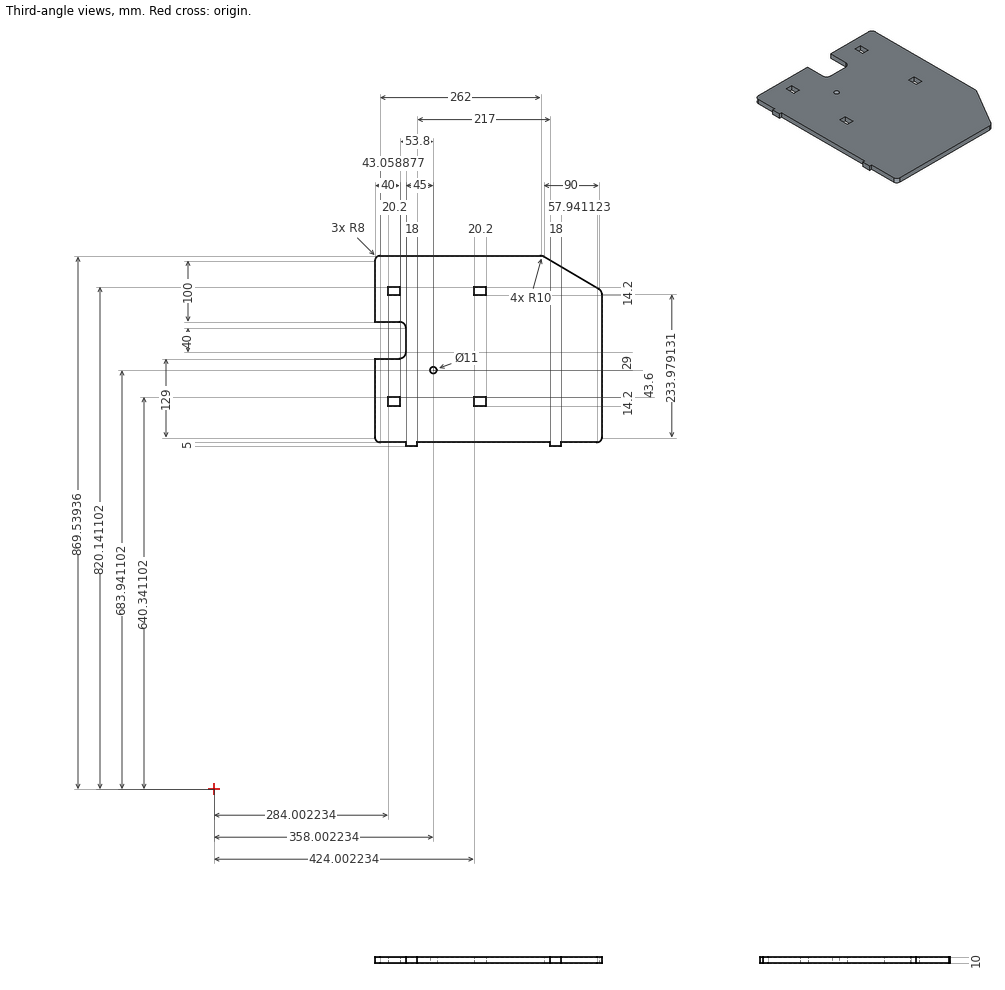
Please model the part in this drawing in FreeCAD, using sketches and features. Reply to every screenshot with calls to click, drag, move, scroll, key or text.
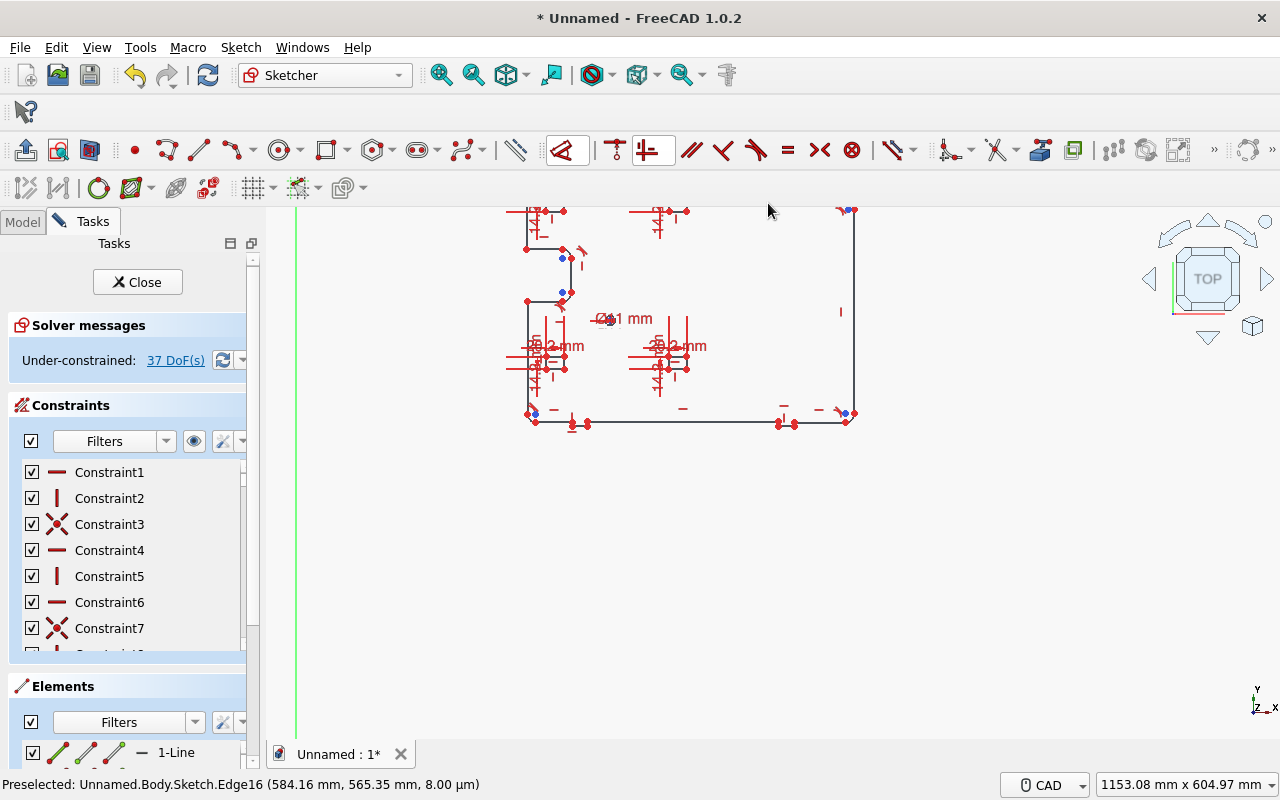
scroll(810, 421, down, 4)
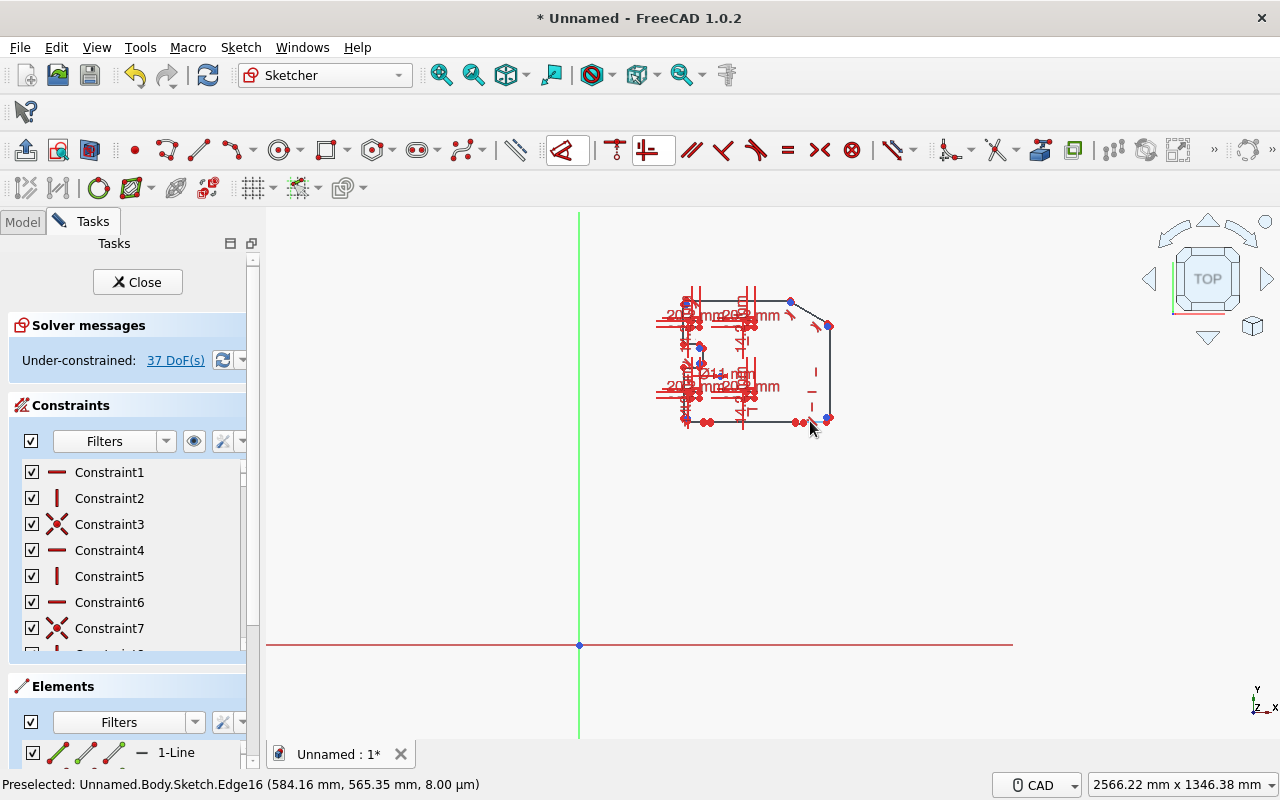
scroll(791, 301, up, 12)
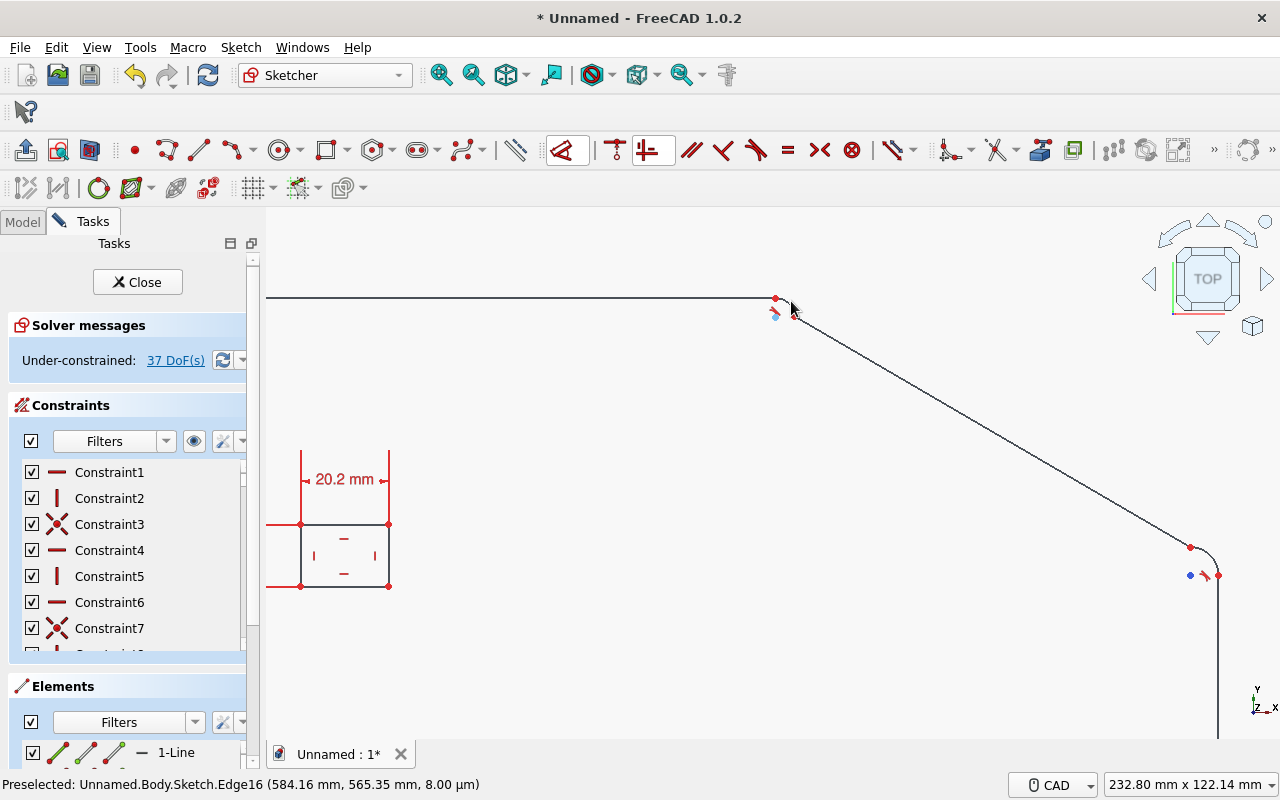
click(789, 303)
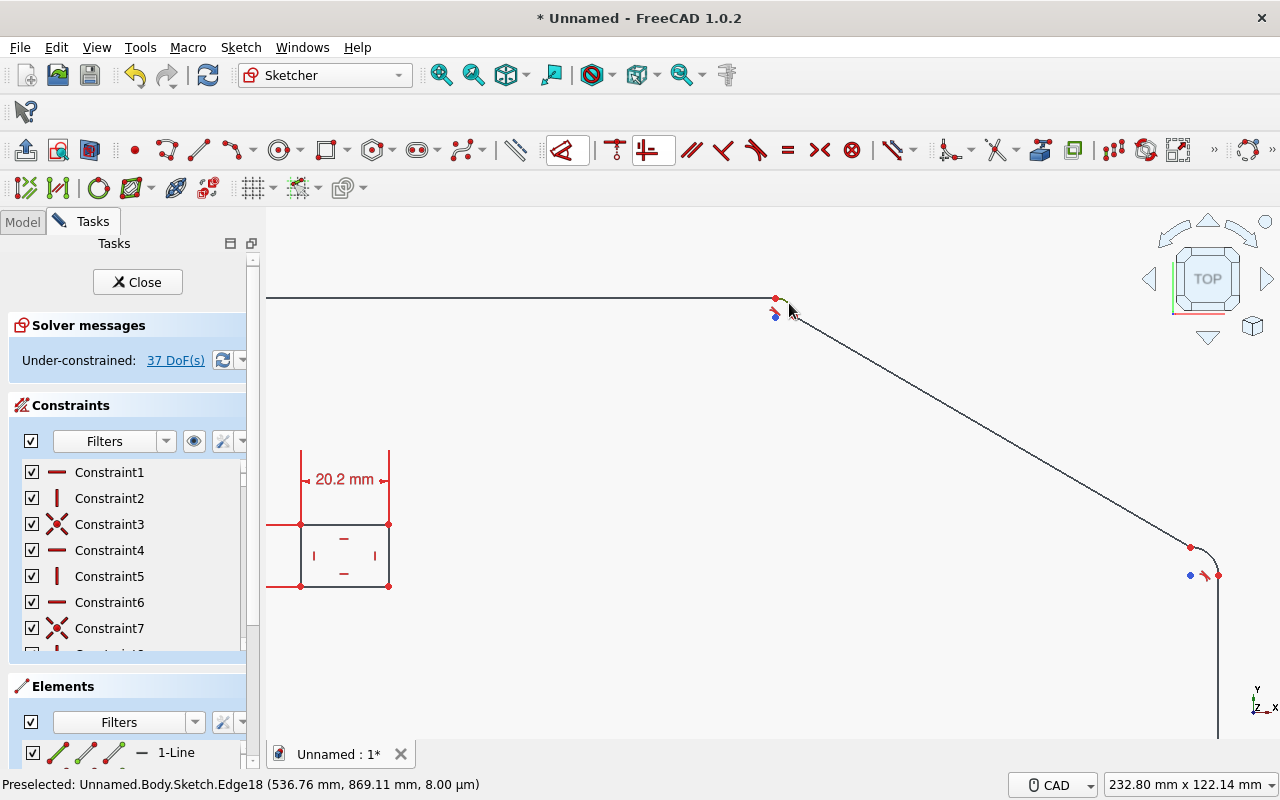
scroll(791, 301, down, 12)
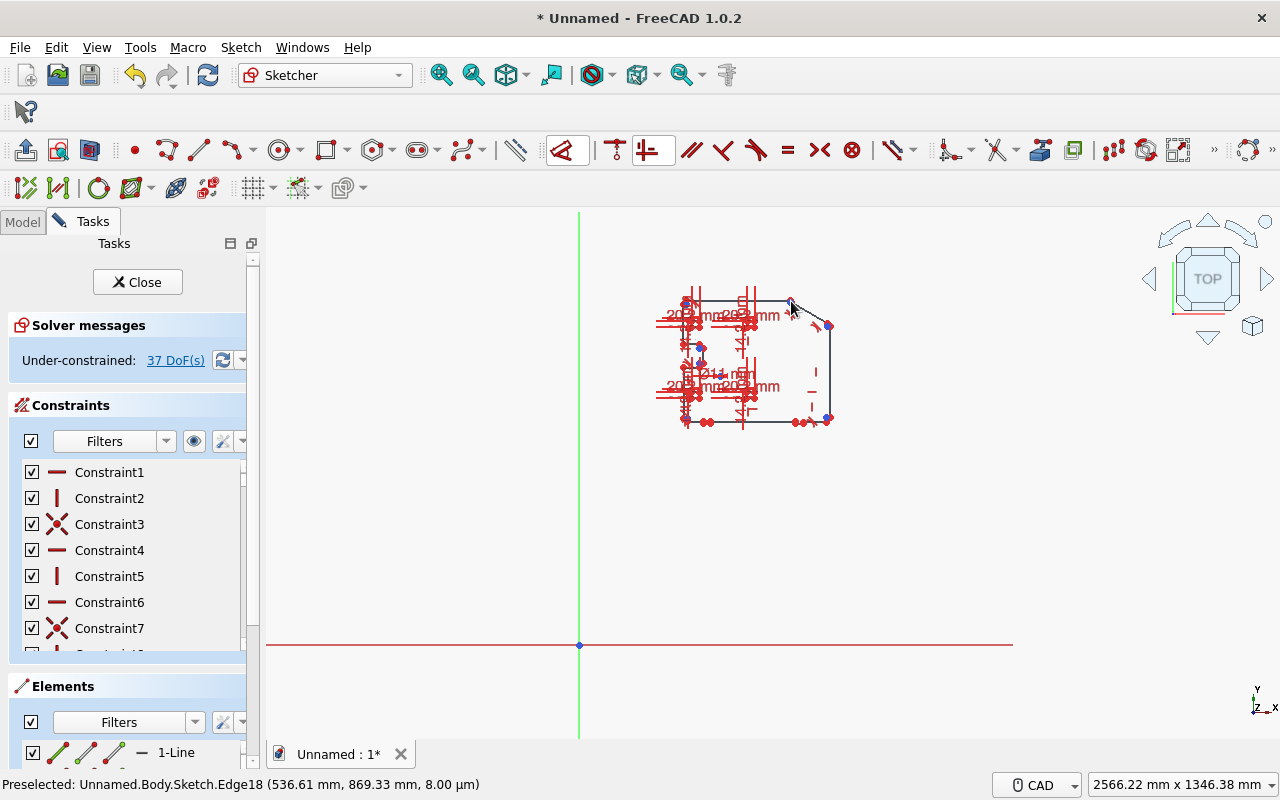
scroll(703, 346, up, 11)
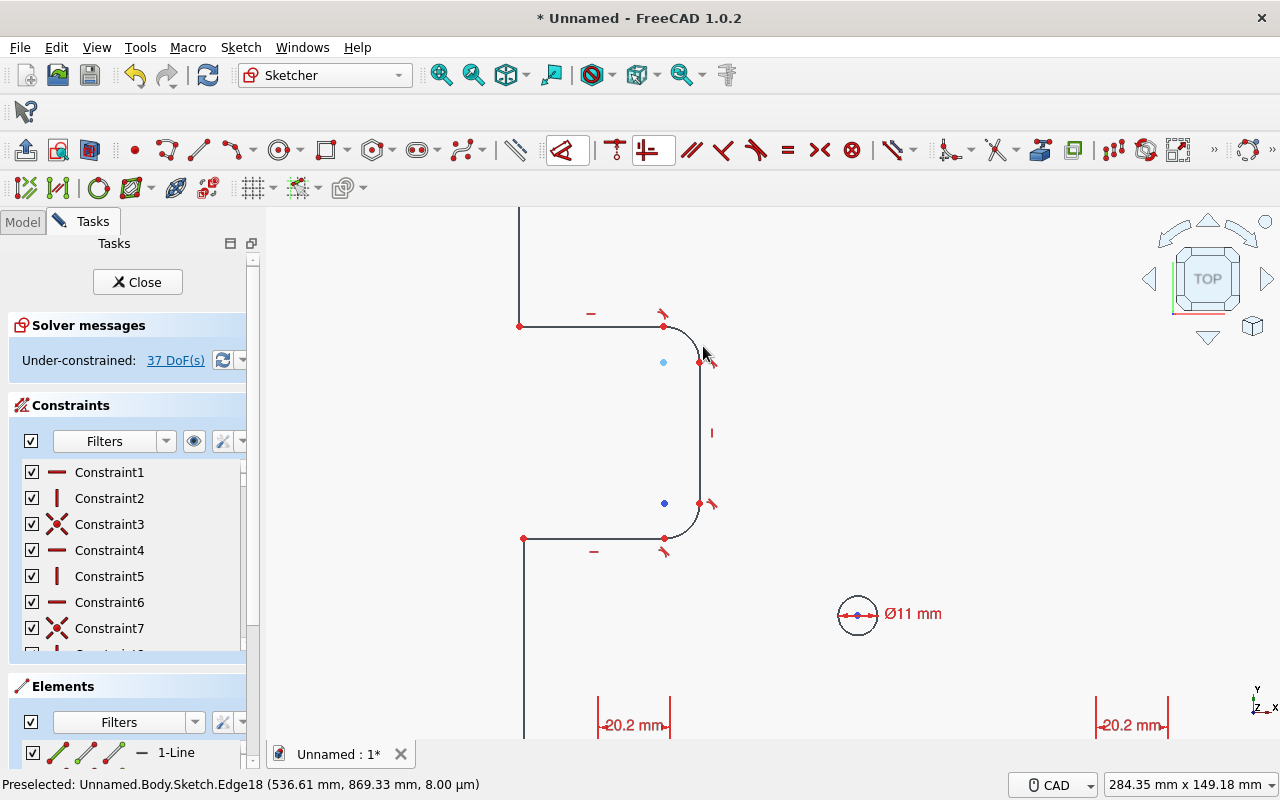
click(696, 346)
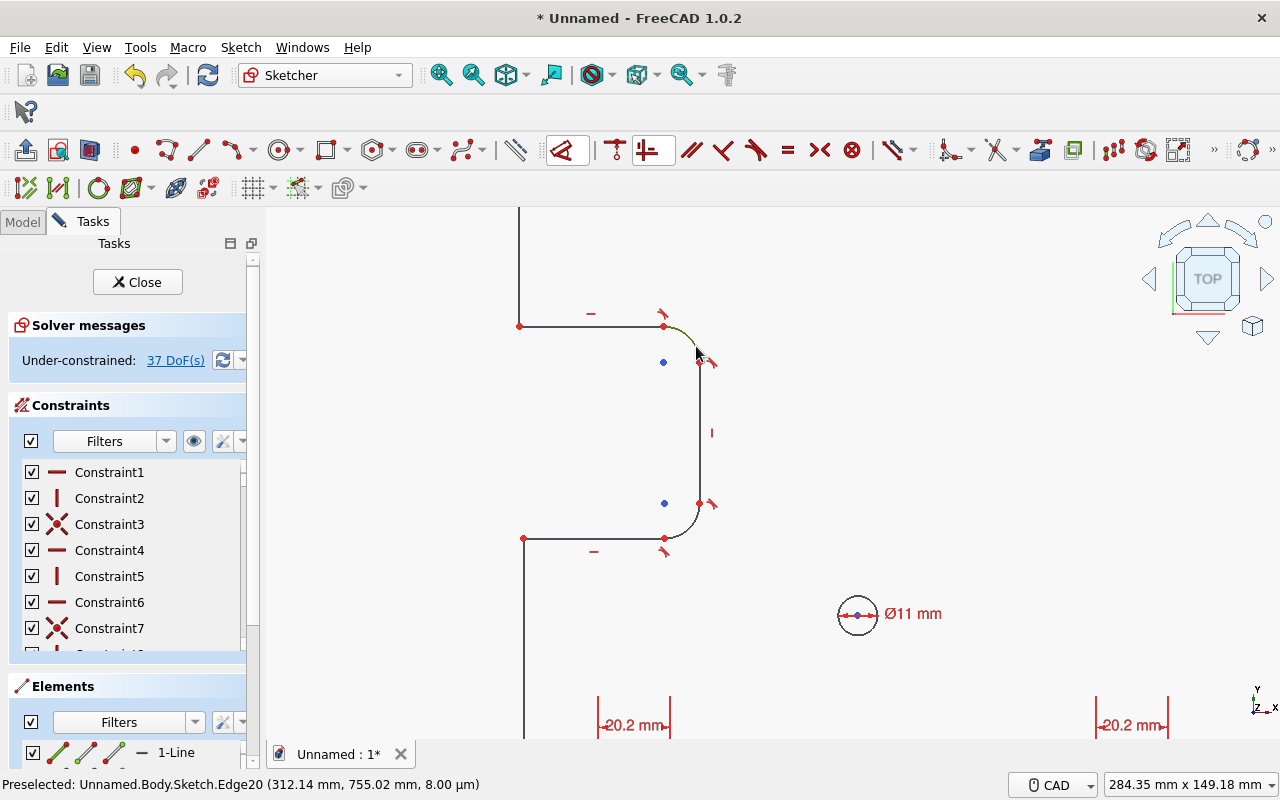
click(680, 535)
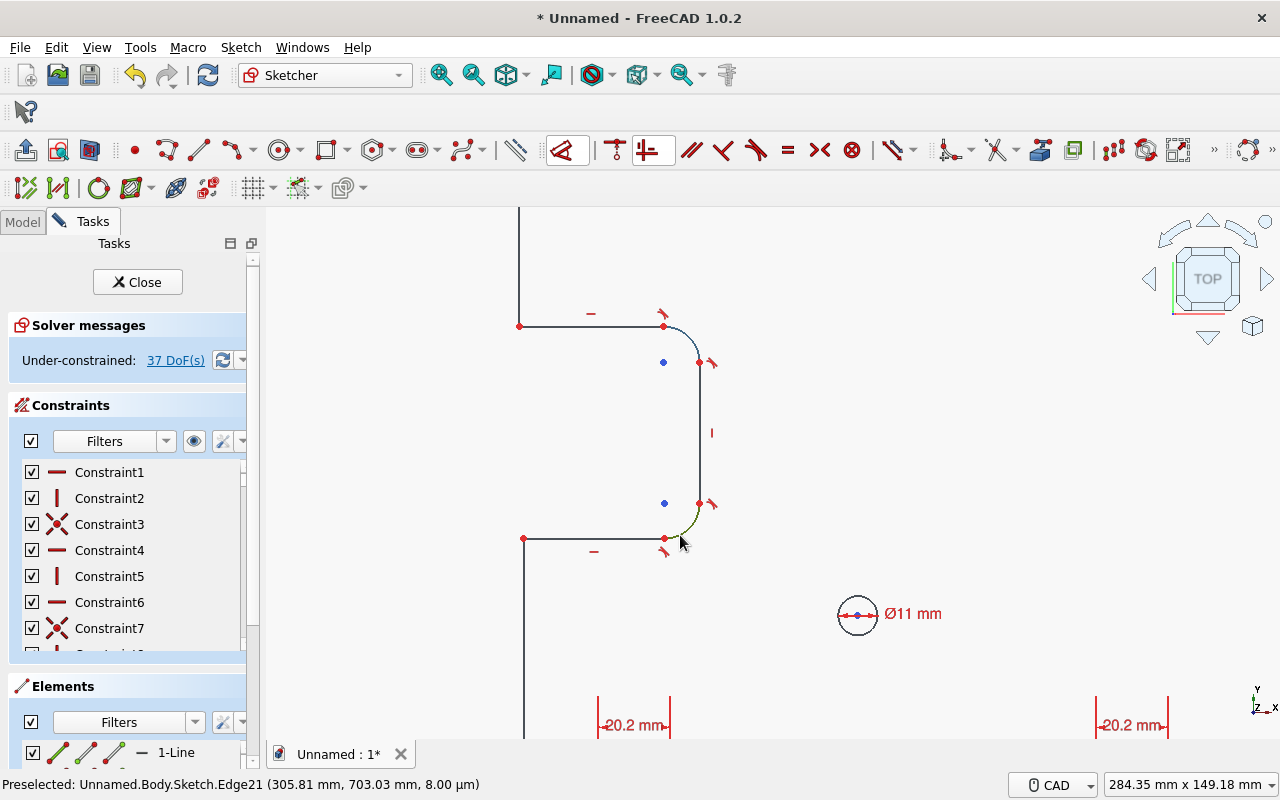
scroll(703, 346, down, 11)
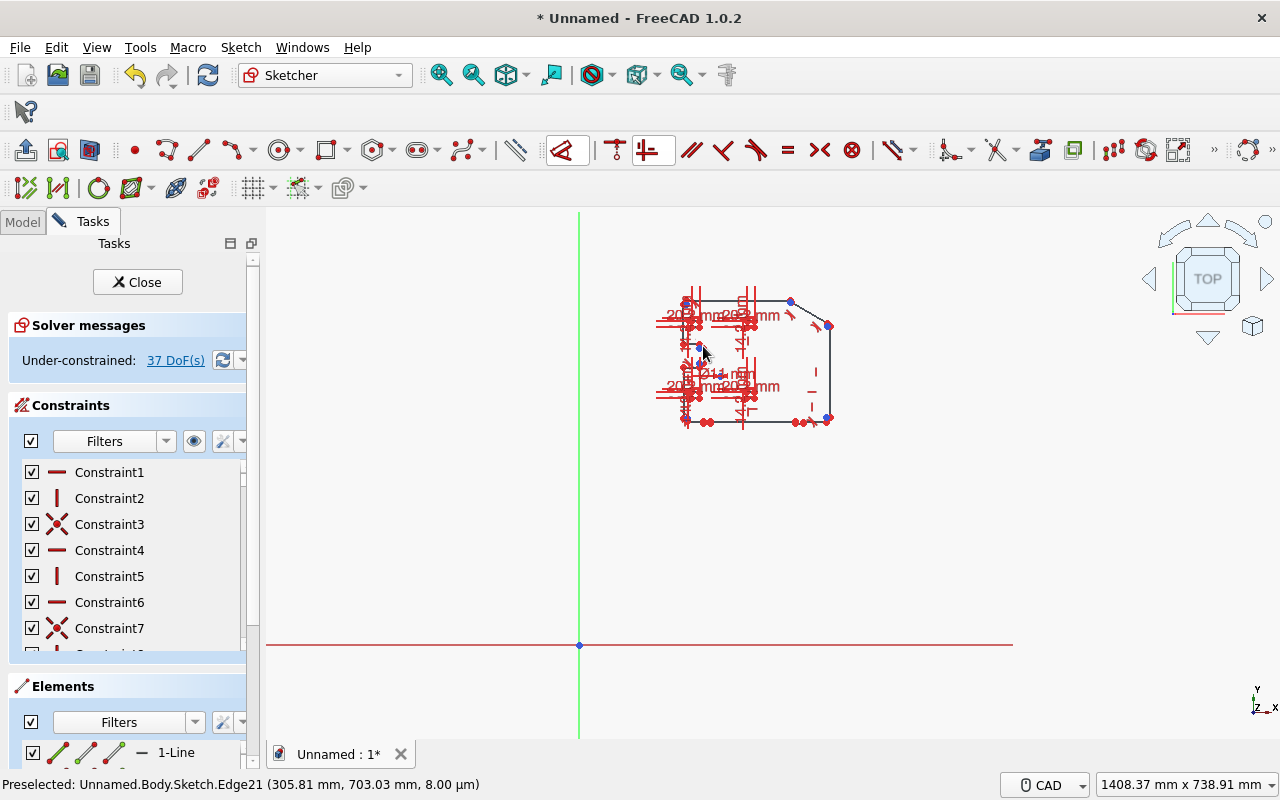
scroll(830, 325, up, 13)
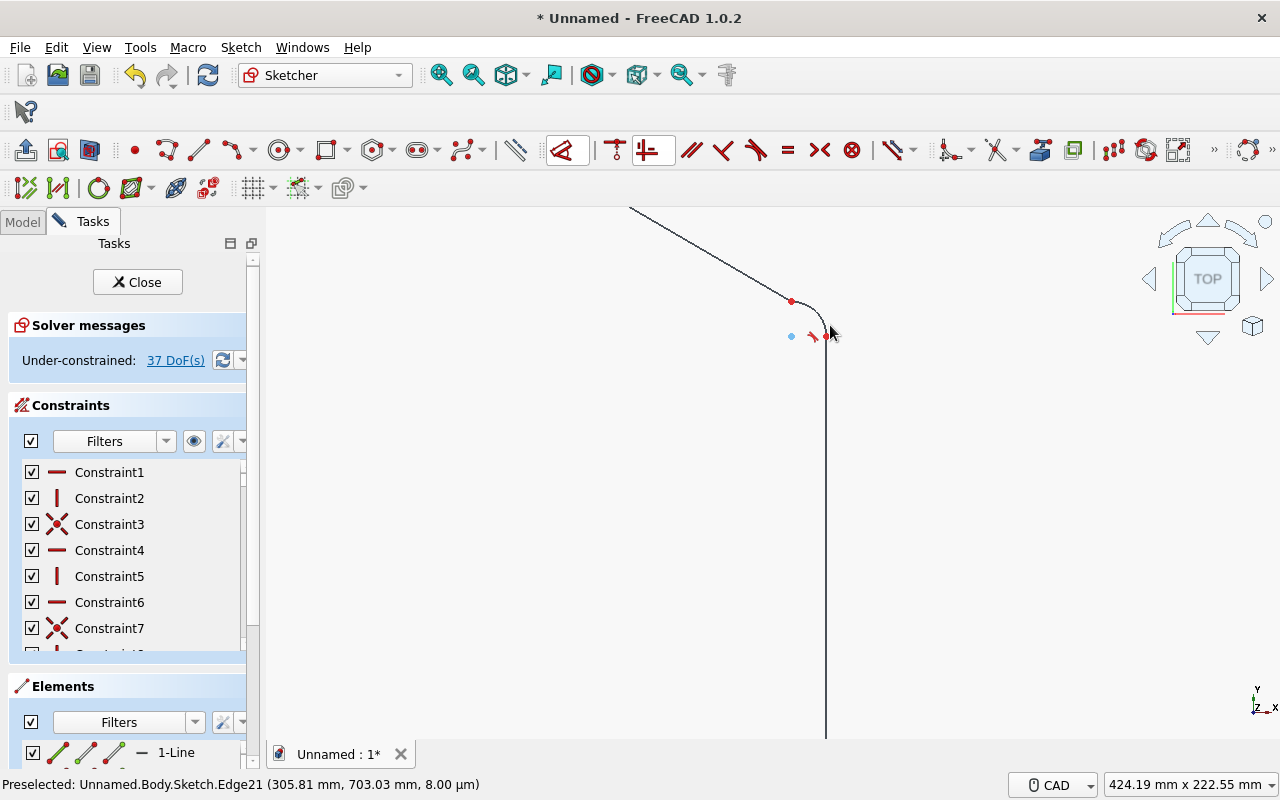
click(823, 321)